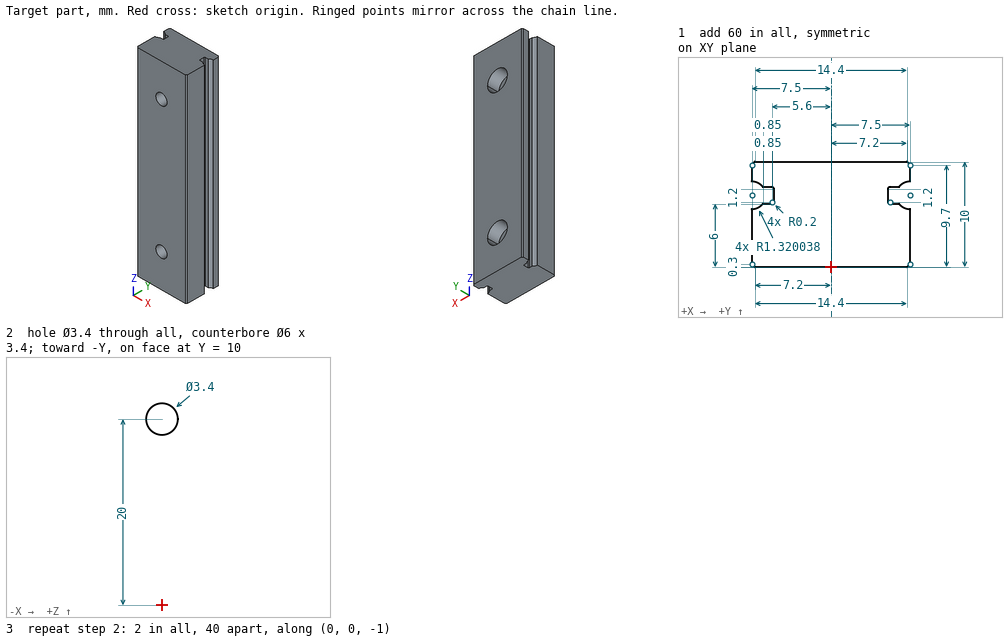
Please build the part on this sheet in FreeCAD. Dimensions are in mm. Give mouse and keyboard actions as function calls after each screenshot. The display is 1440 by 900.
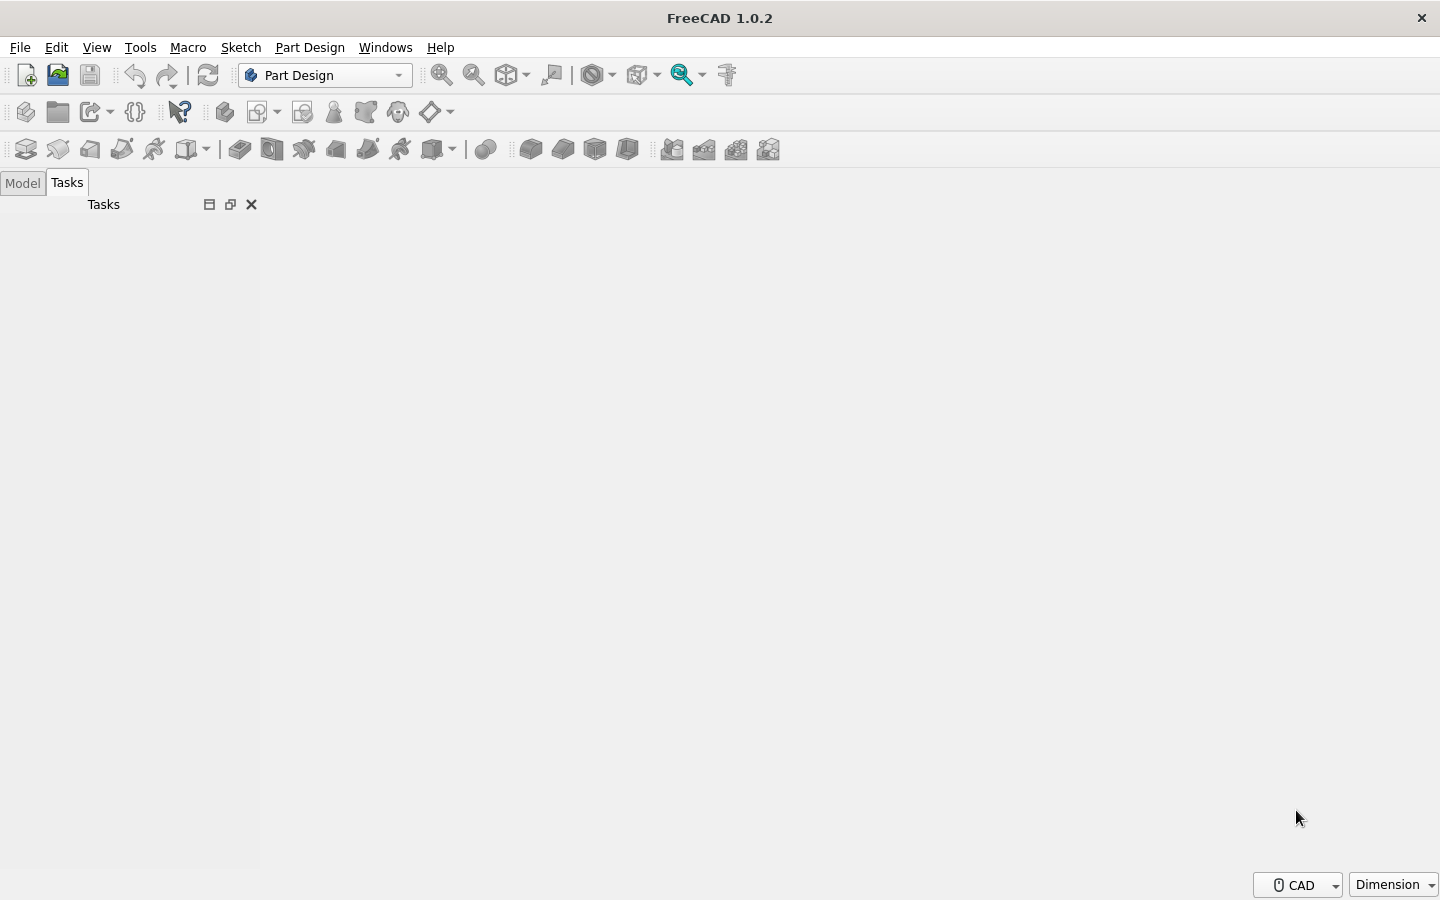
click(26, 76)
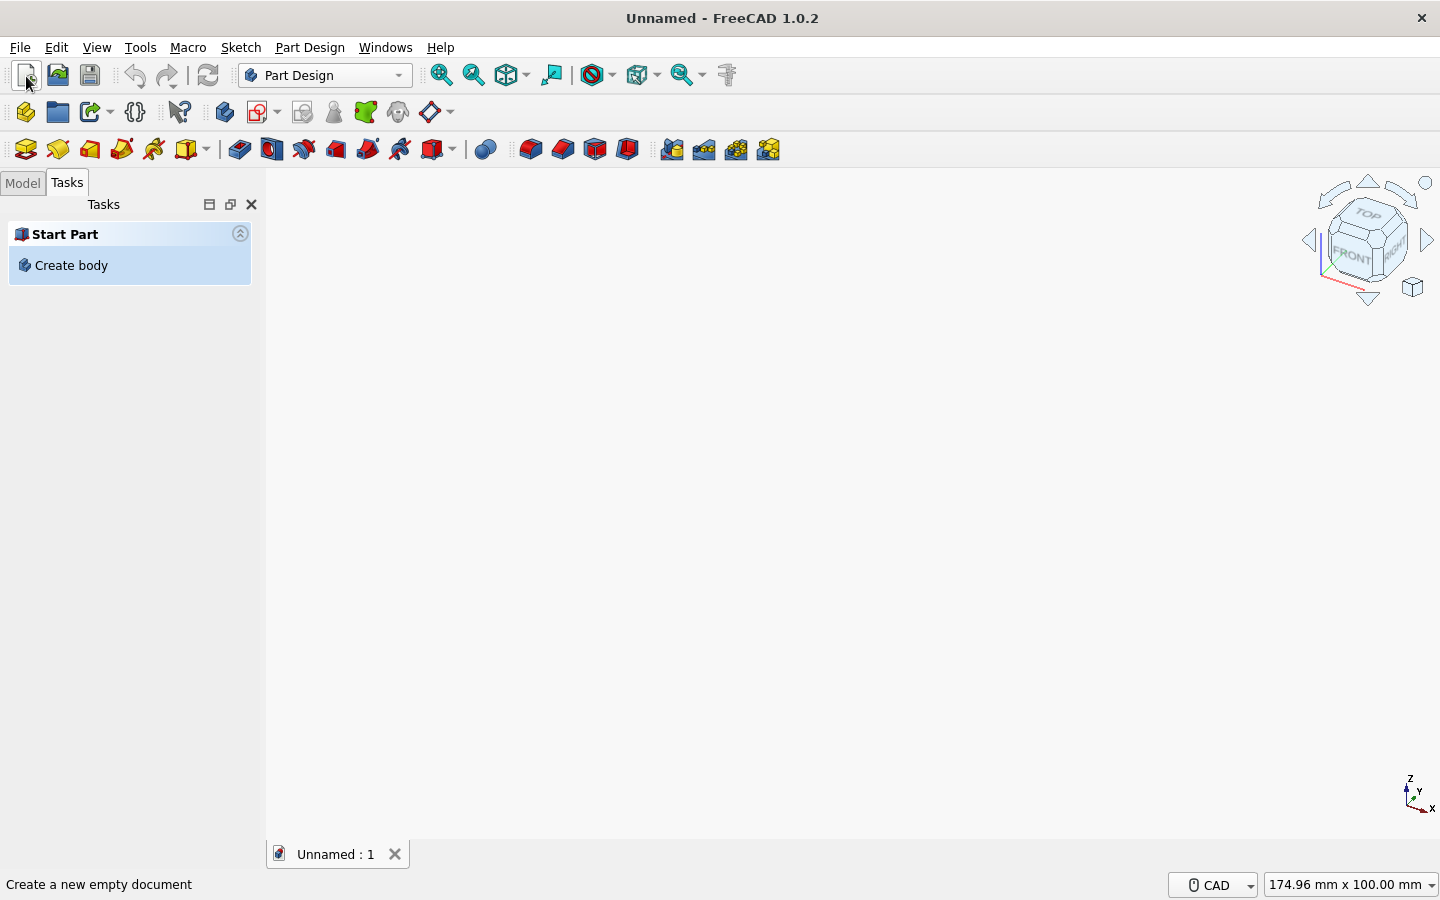
click(258, 112)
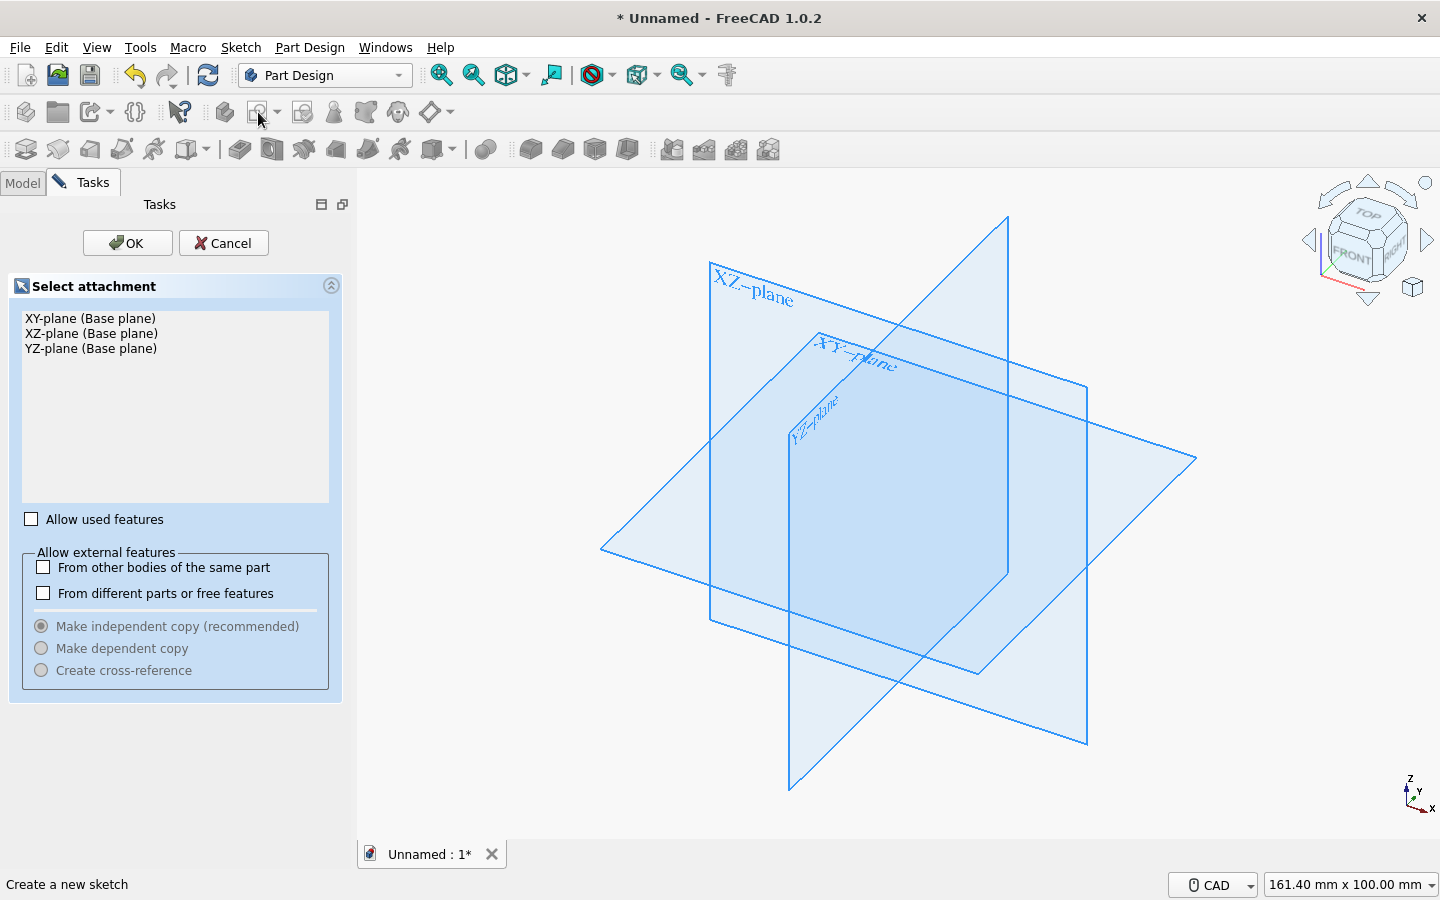
click(82, 318)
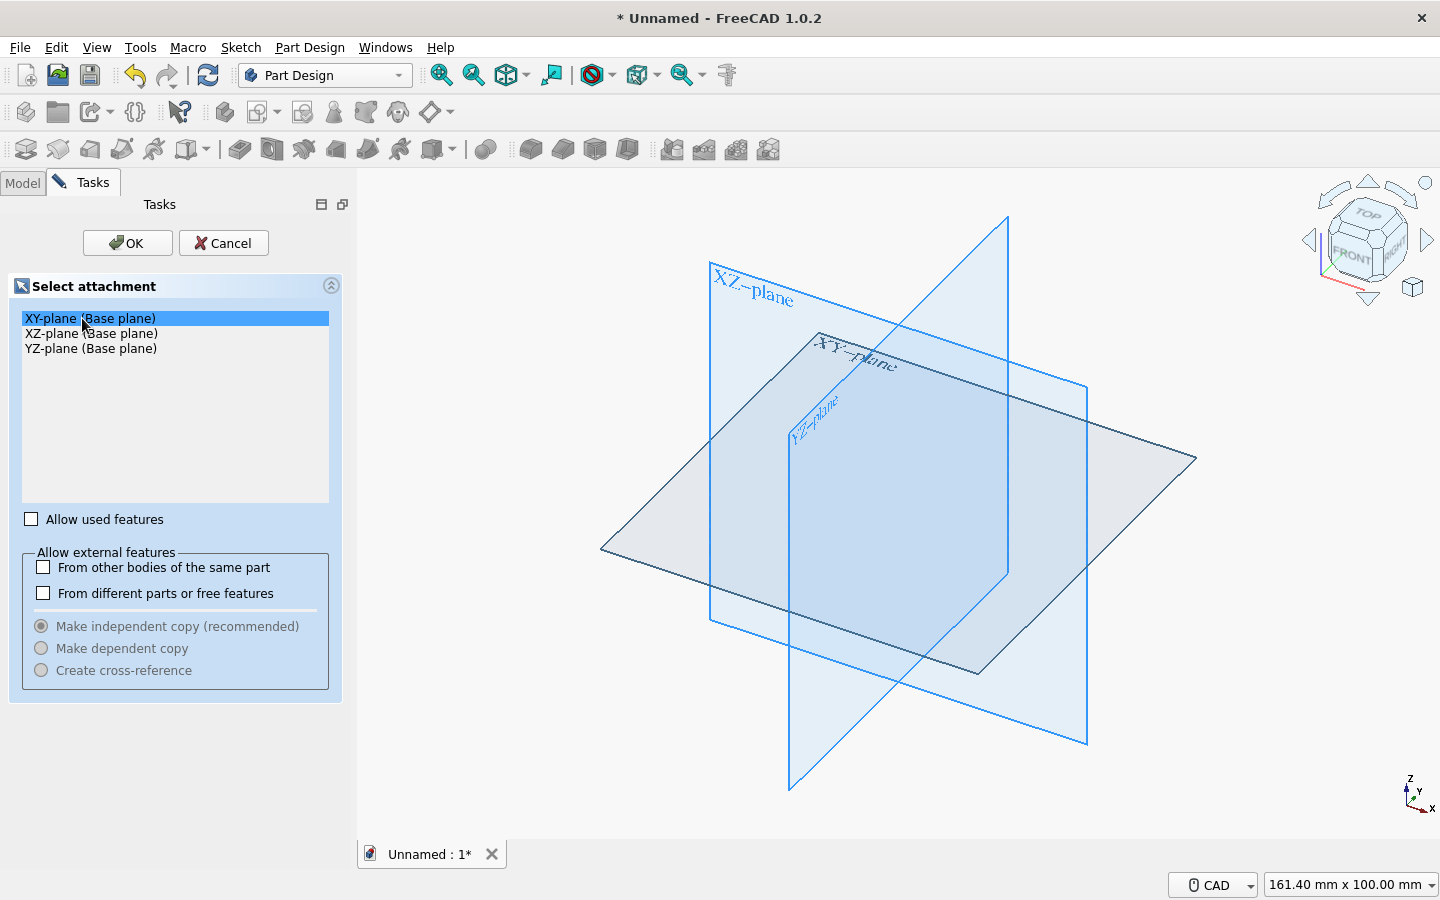
click(128, 243)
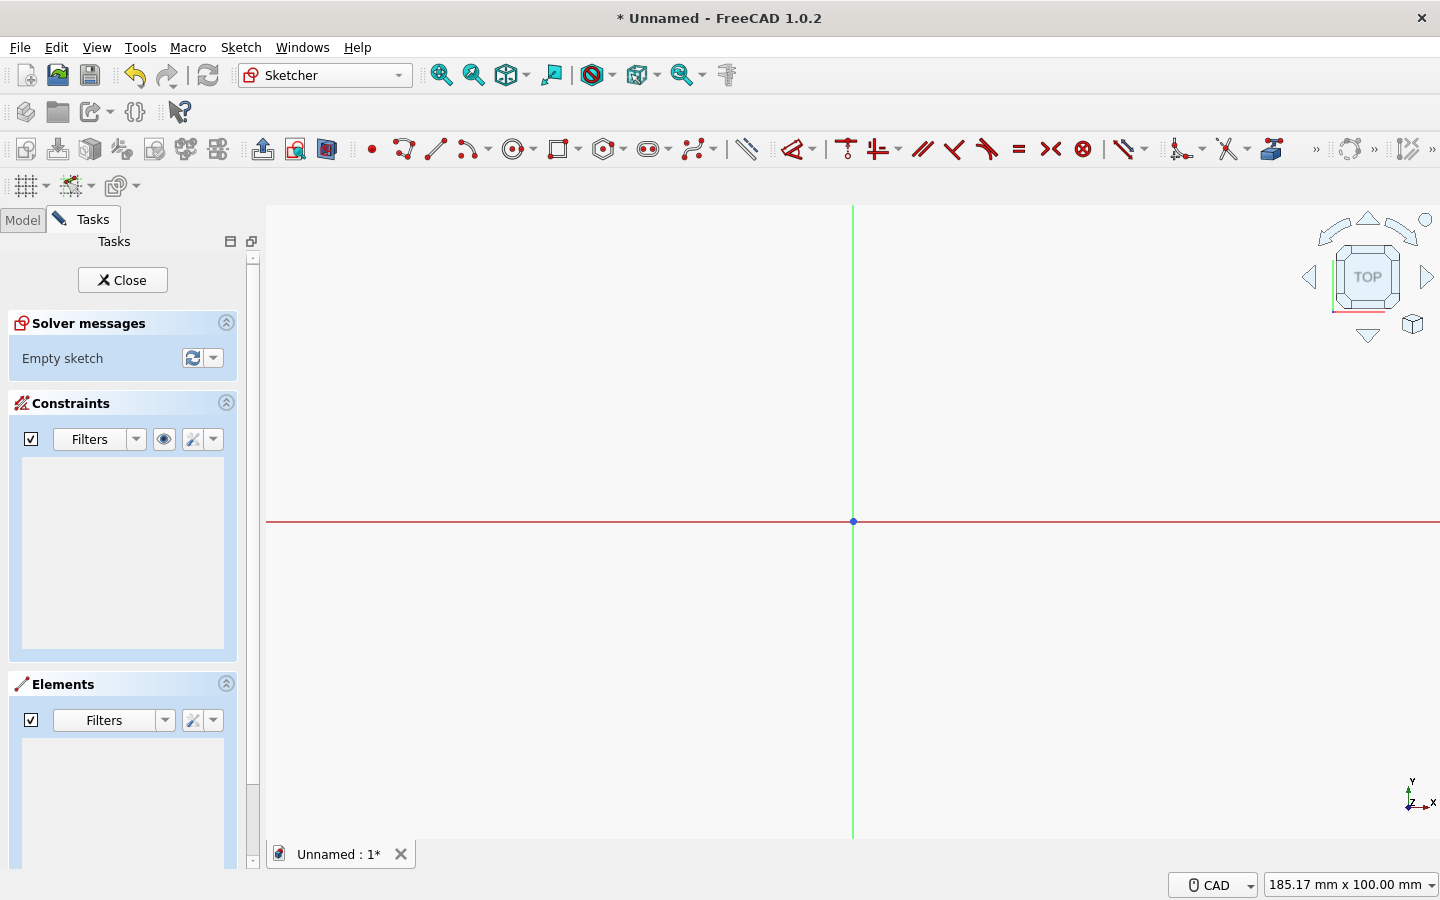
scroll(867, 484, up, 9)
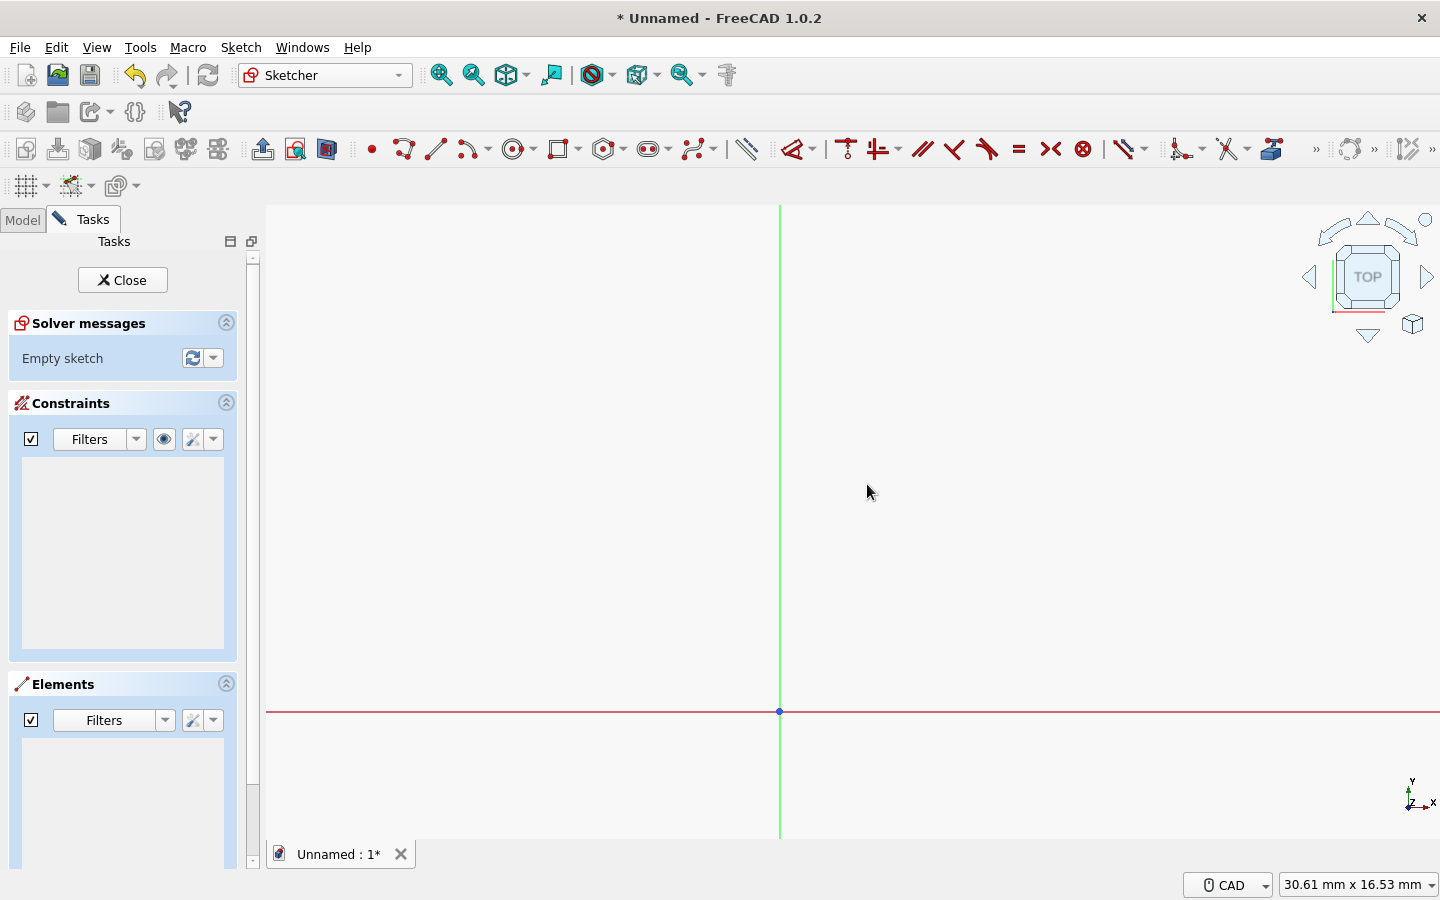
click(436, 150)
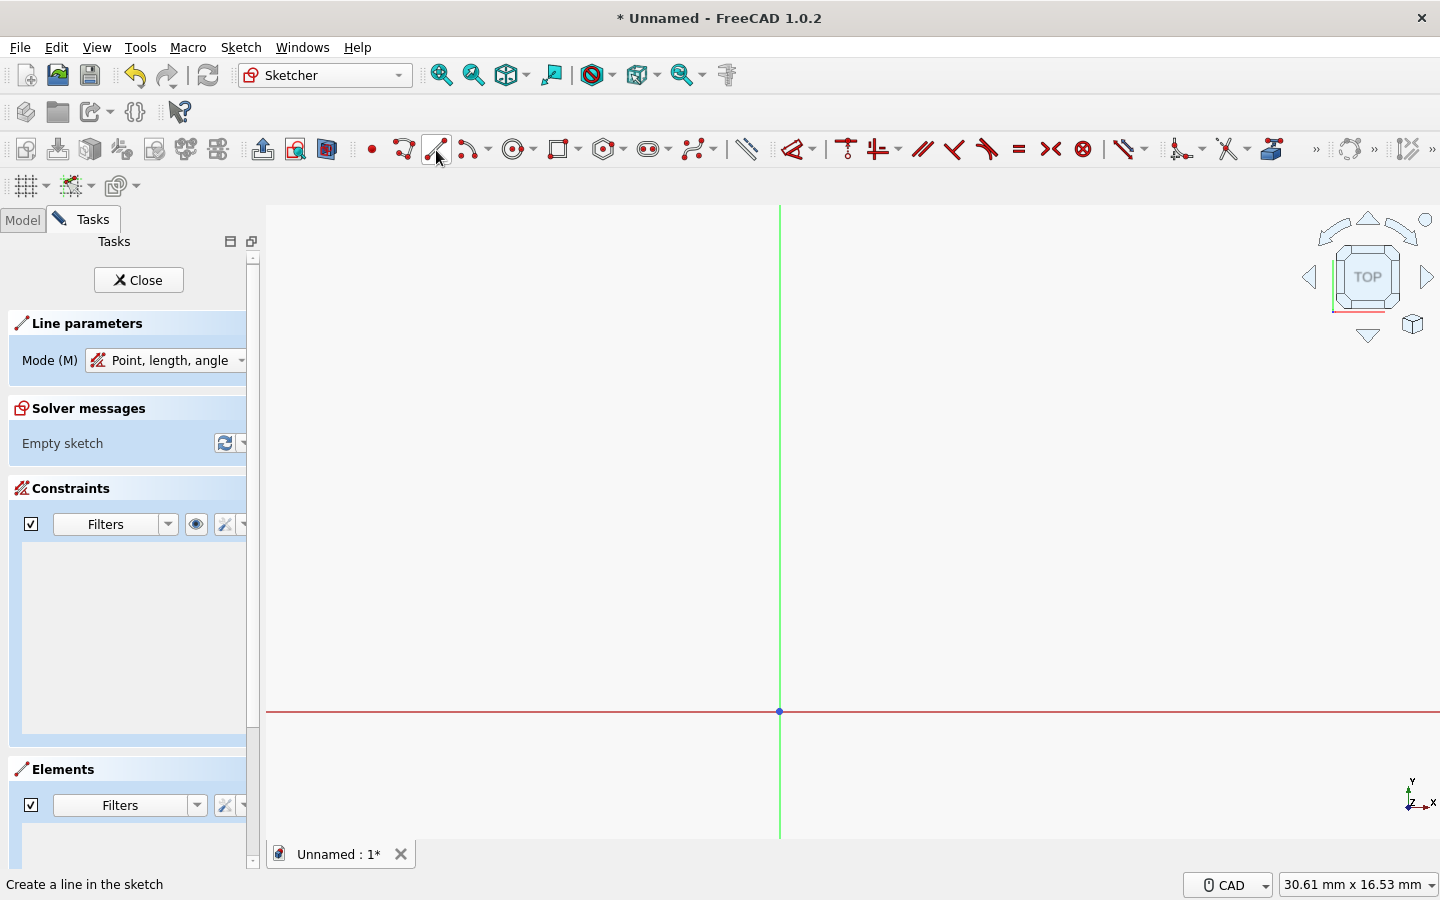
click(532, 420)
click(565, 420)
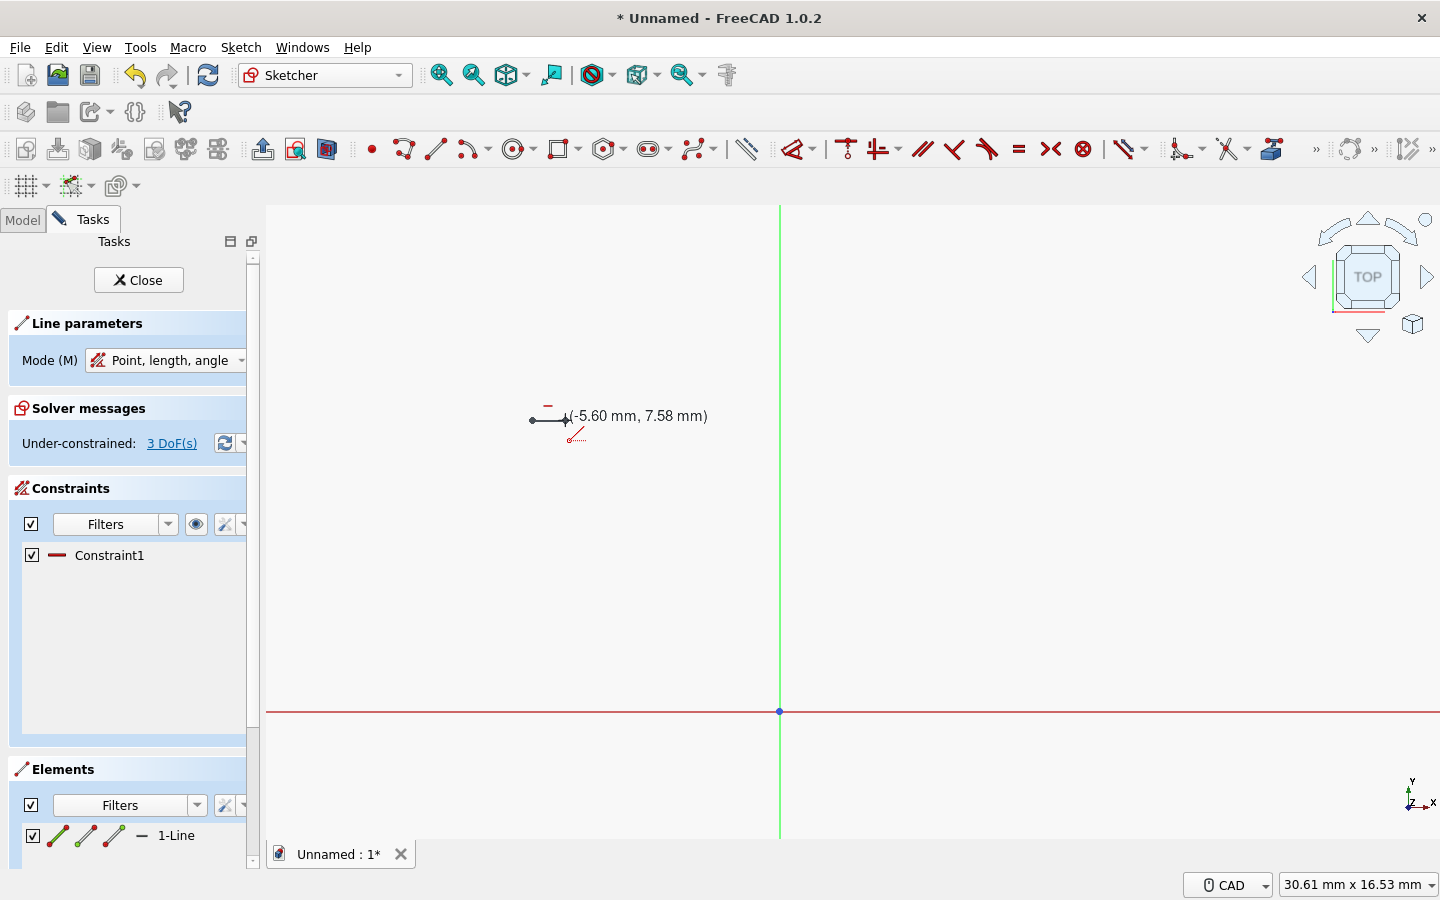
scroll(573, 428, up, 2)